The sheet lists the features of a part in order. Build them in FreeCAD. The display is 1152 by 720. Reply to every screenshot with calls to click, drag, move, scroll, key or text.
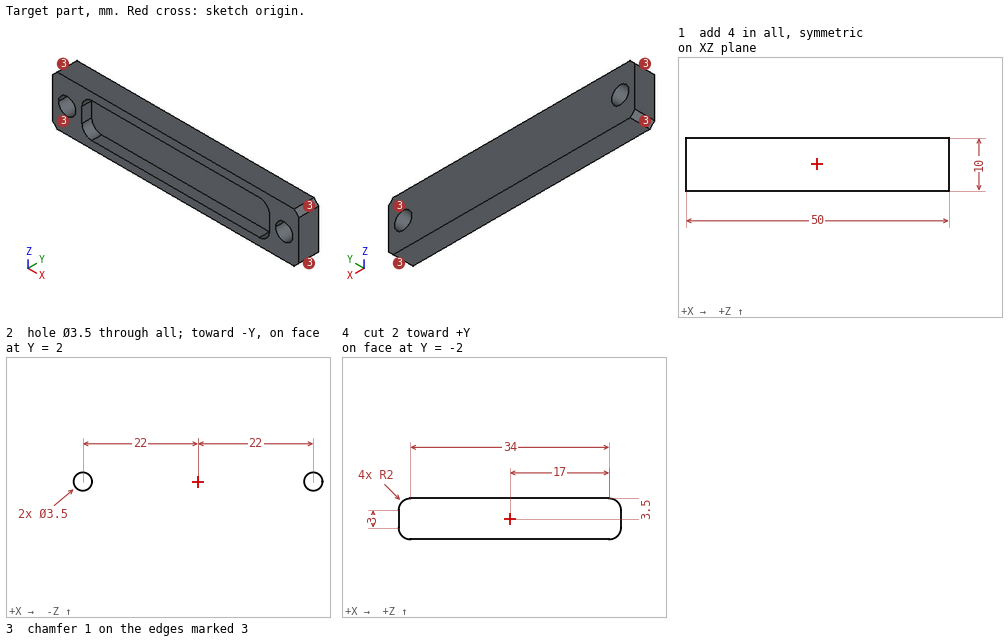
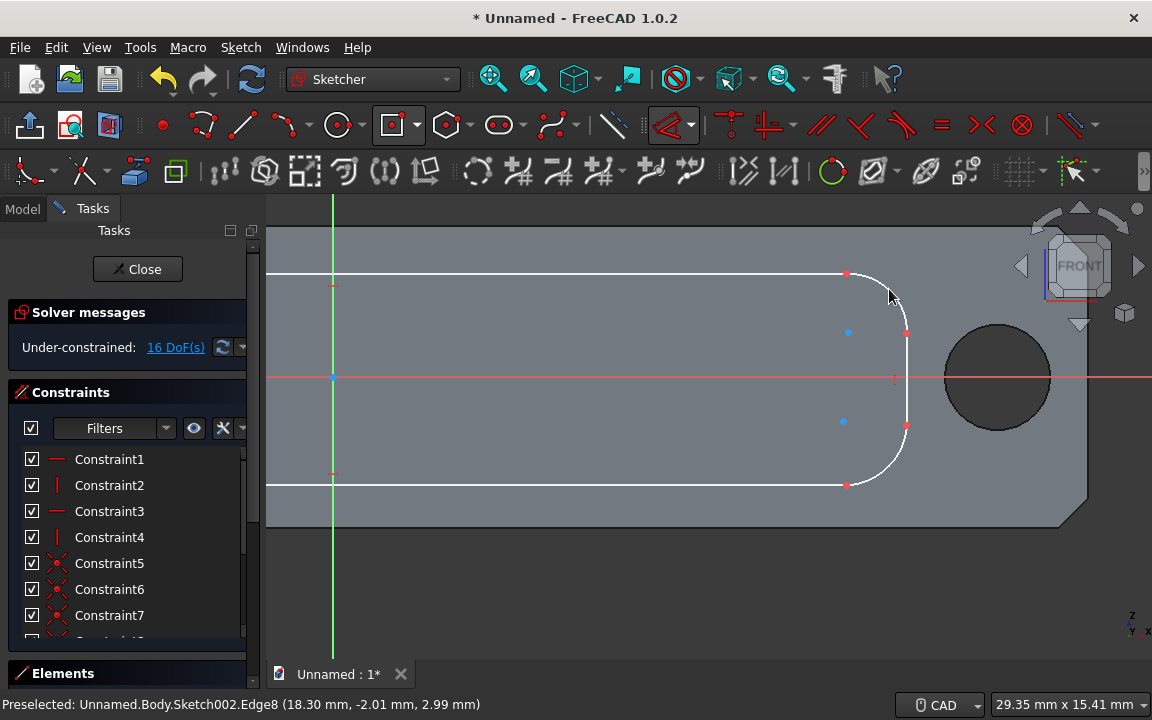
click(539, 274)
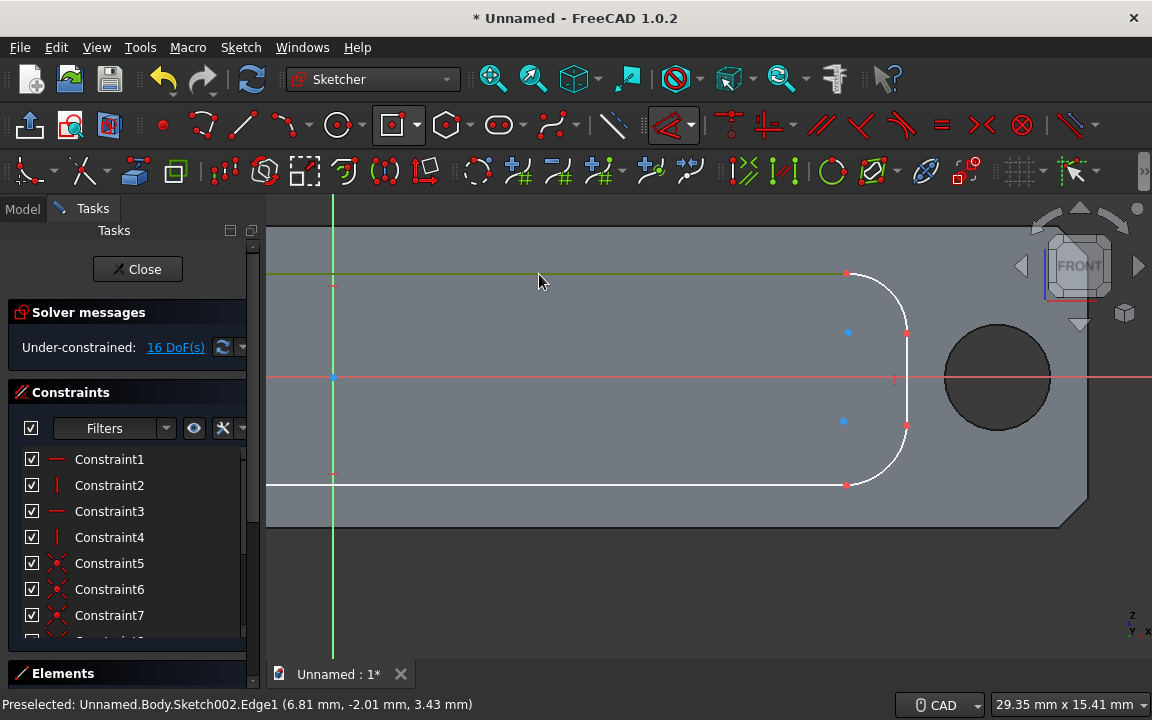
scroll(891, 467, down, 4)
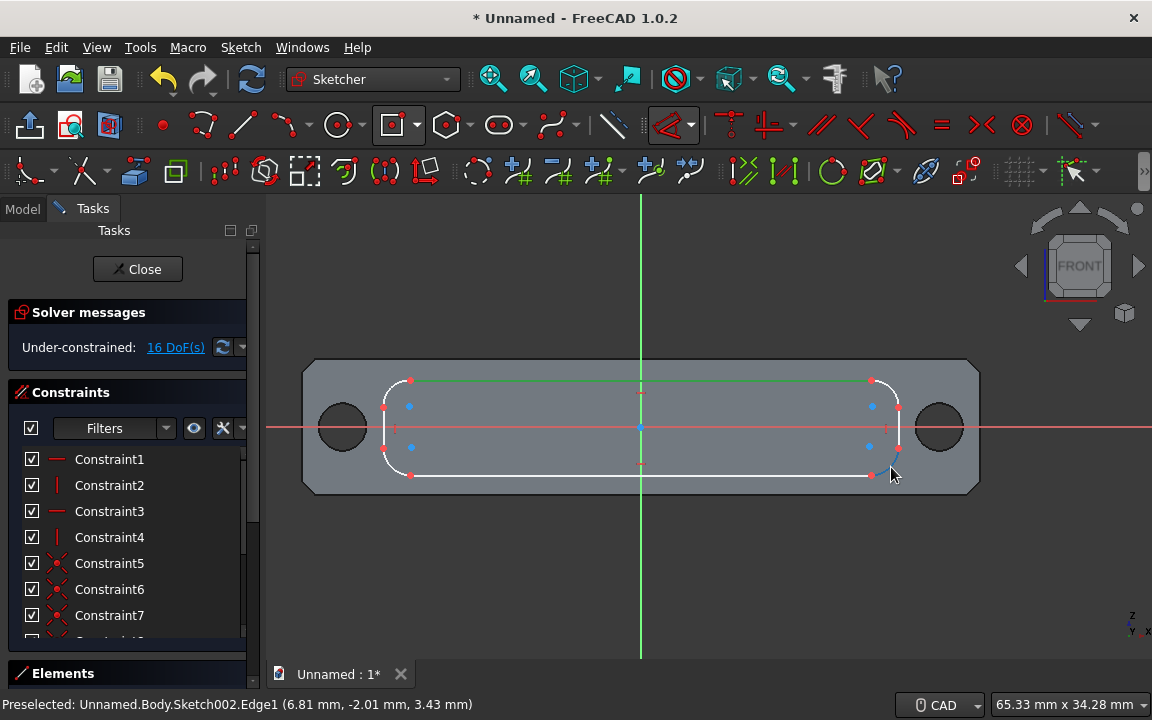
click(398, 383)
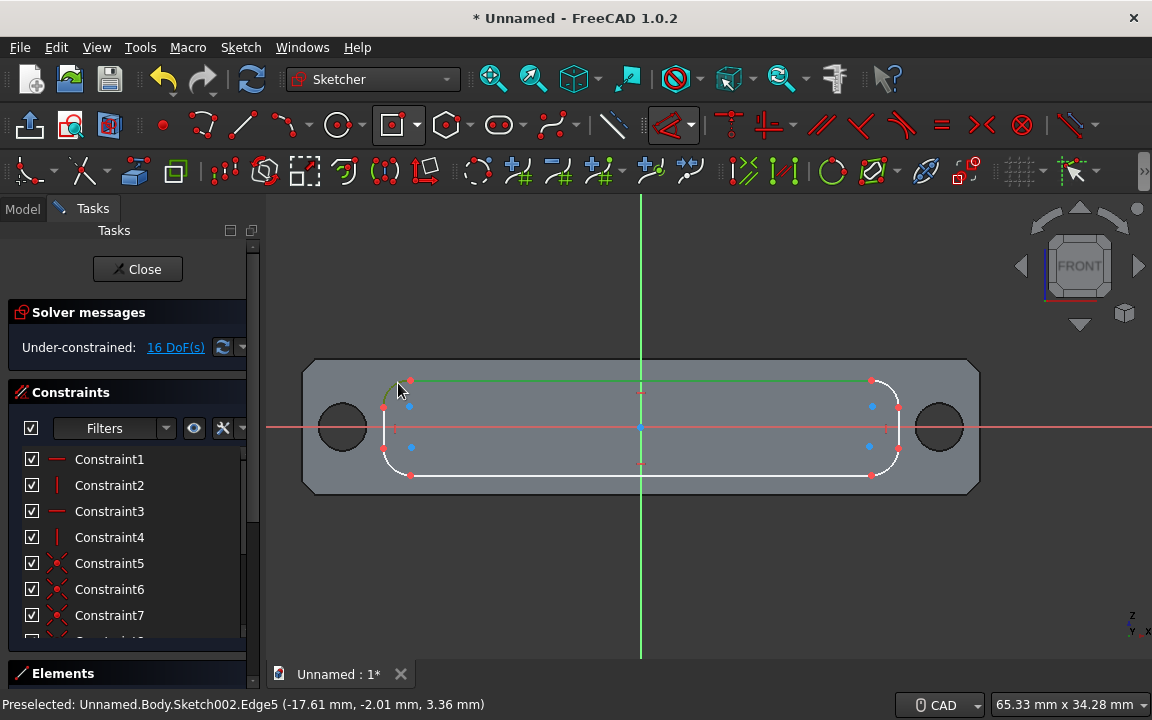
click(902, 126)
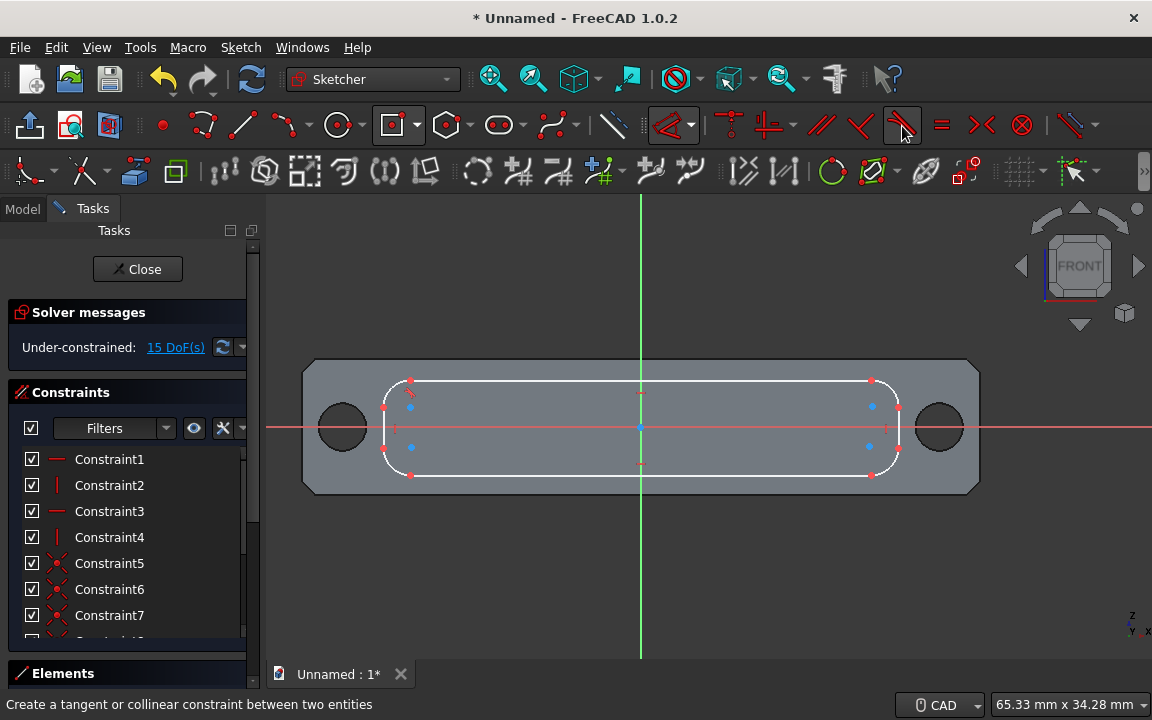
click(733, 381)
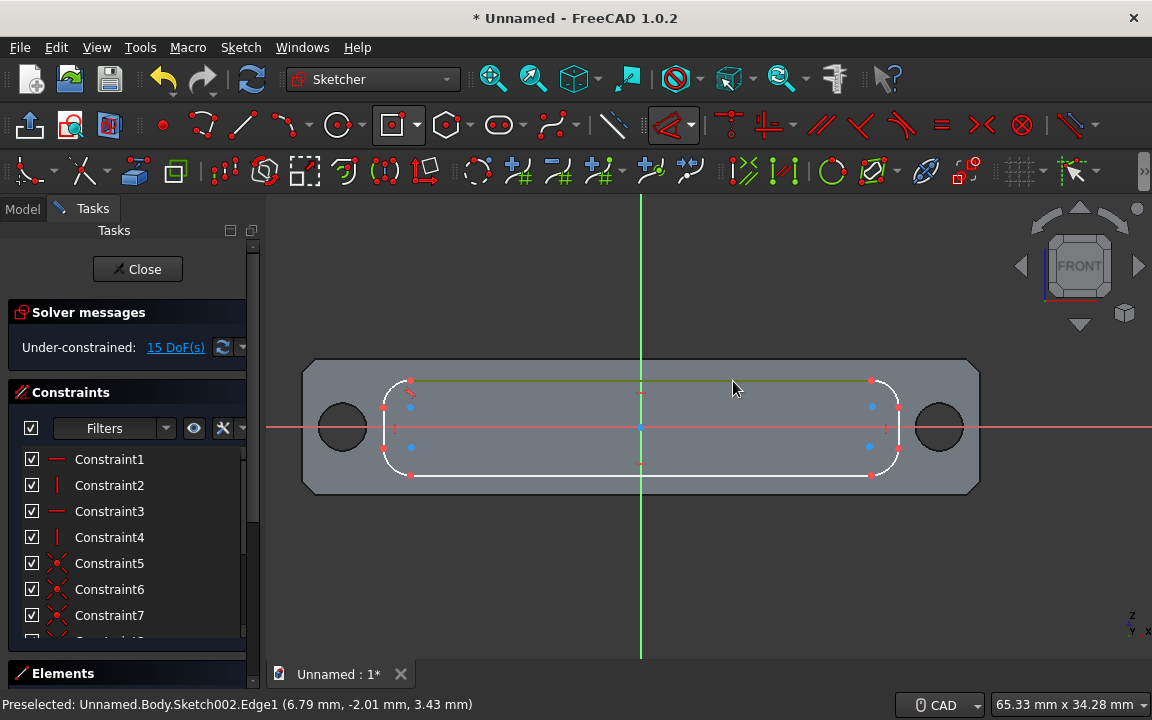
click(896, 395)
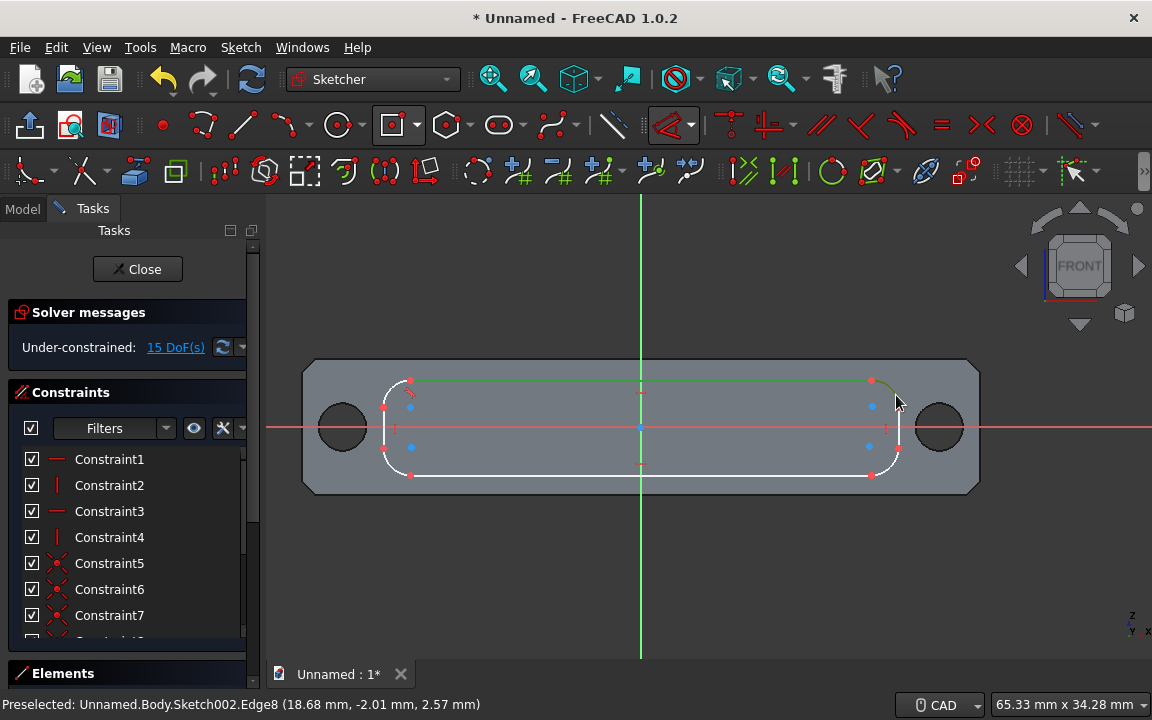
click(902, 126)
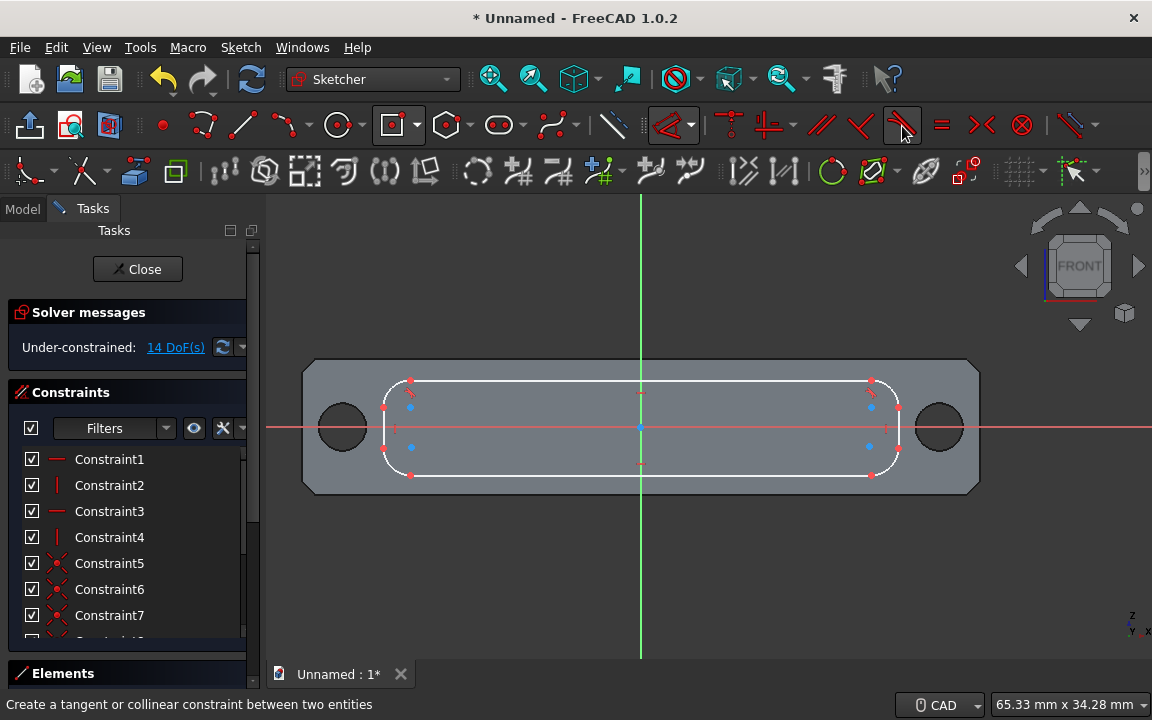
scroll(384, 436, up, 3)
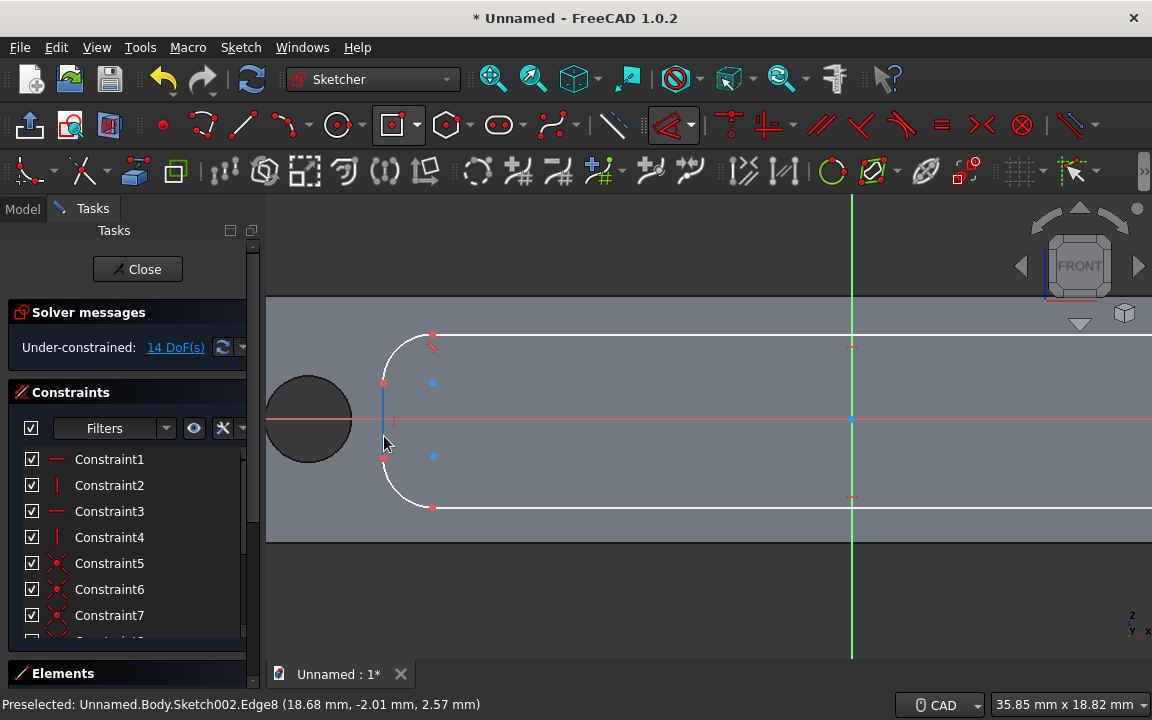
click(383, 436)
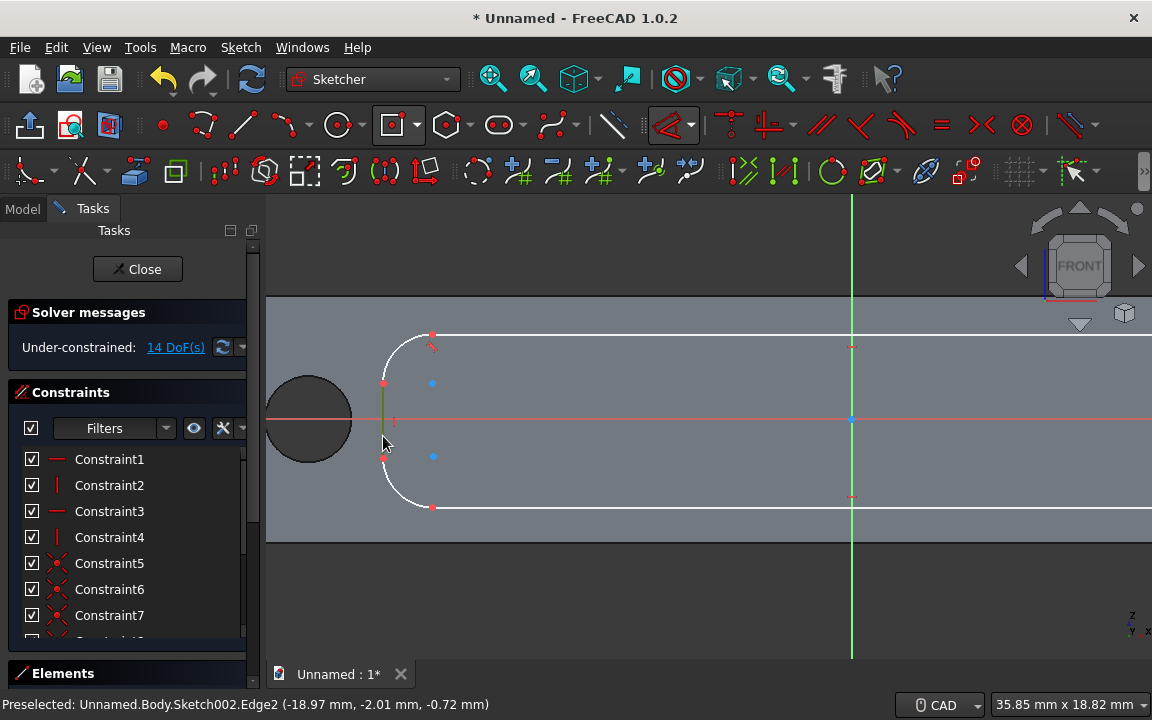
click(410, 340)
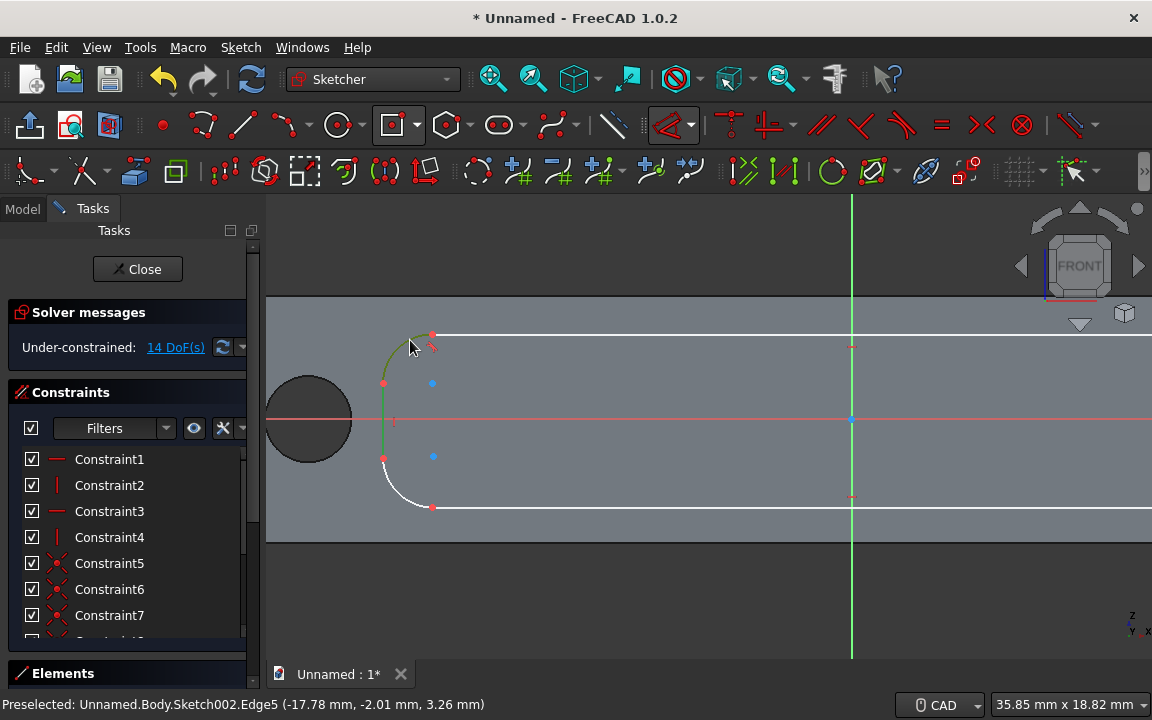
click(902, 126)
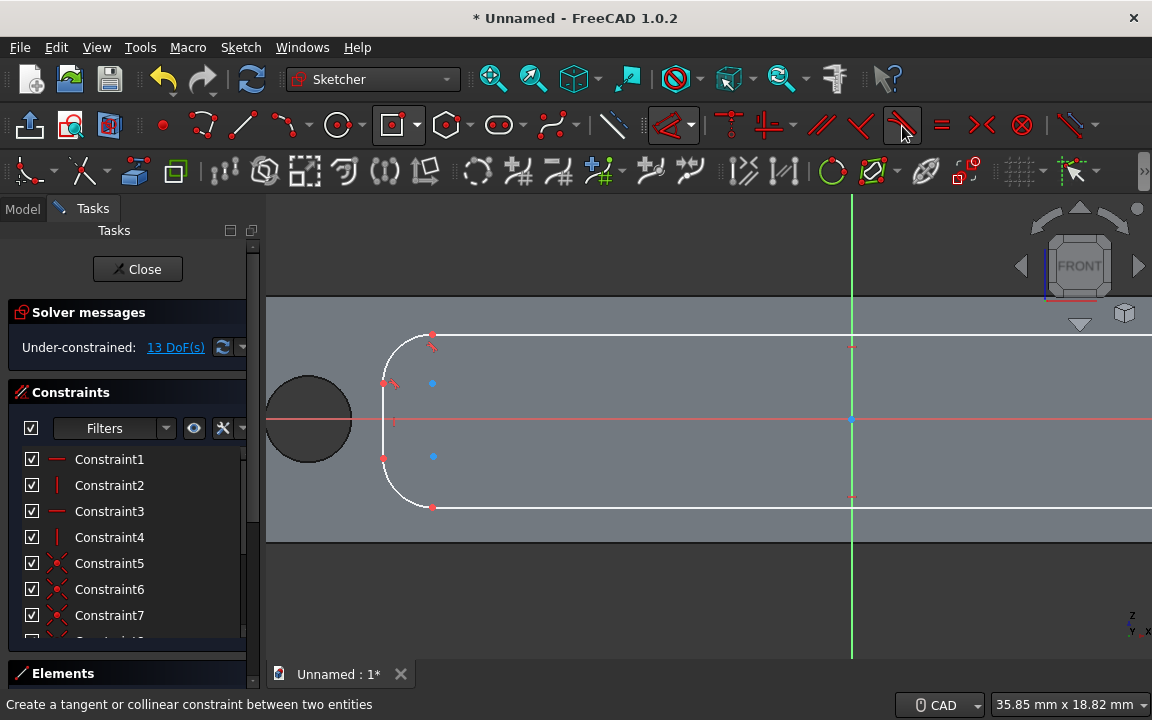
click(383, 406)